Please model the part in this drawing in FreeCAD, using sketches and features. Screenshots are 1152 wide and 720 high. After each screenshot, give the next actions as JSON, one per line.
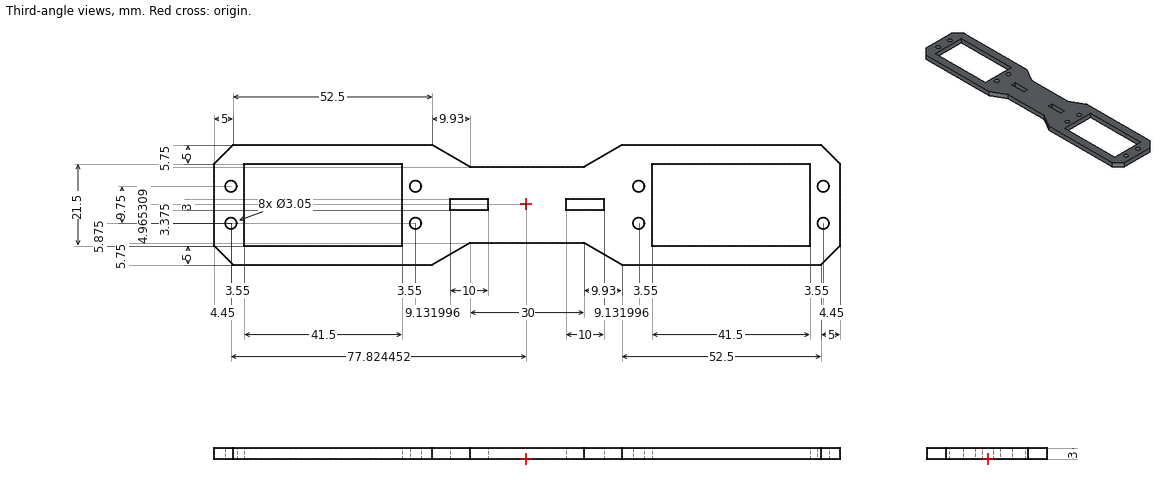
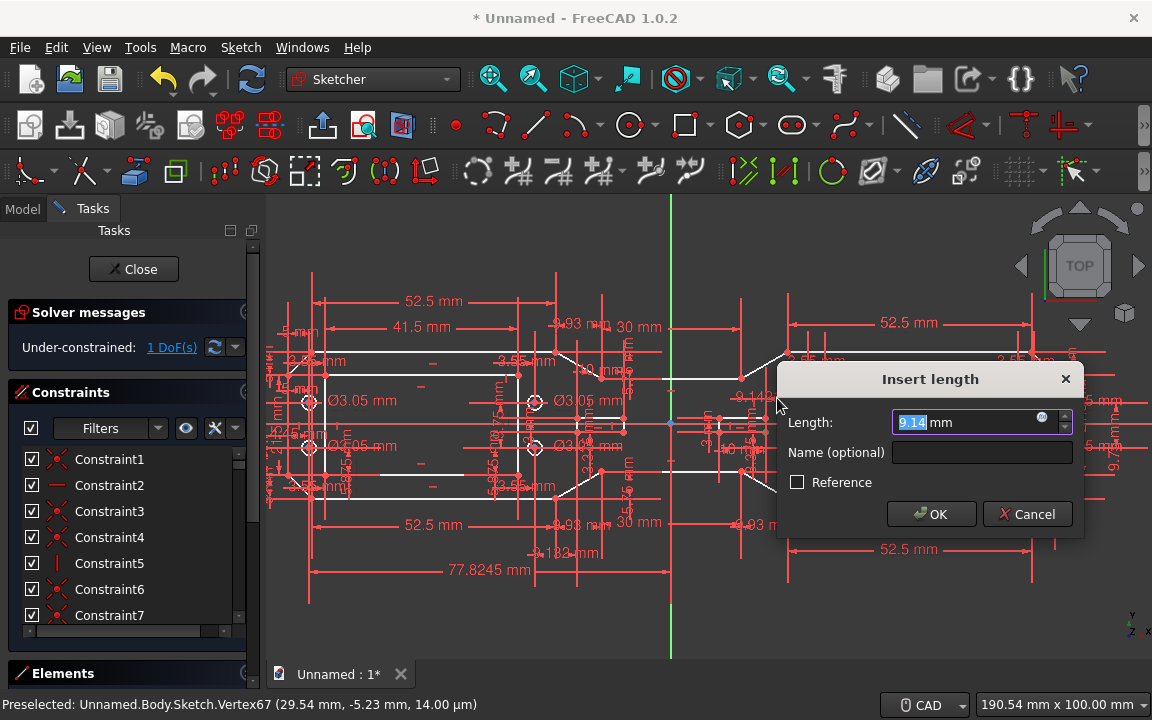
{"action": "type", "text": "9.131996"}
{"action": "key", "text": "Return"}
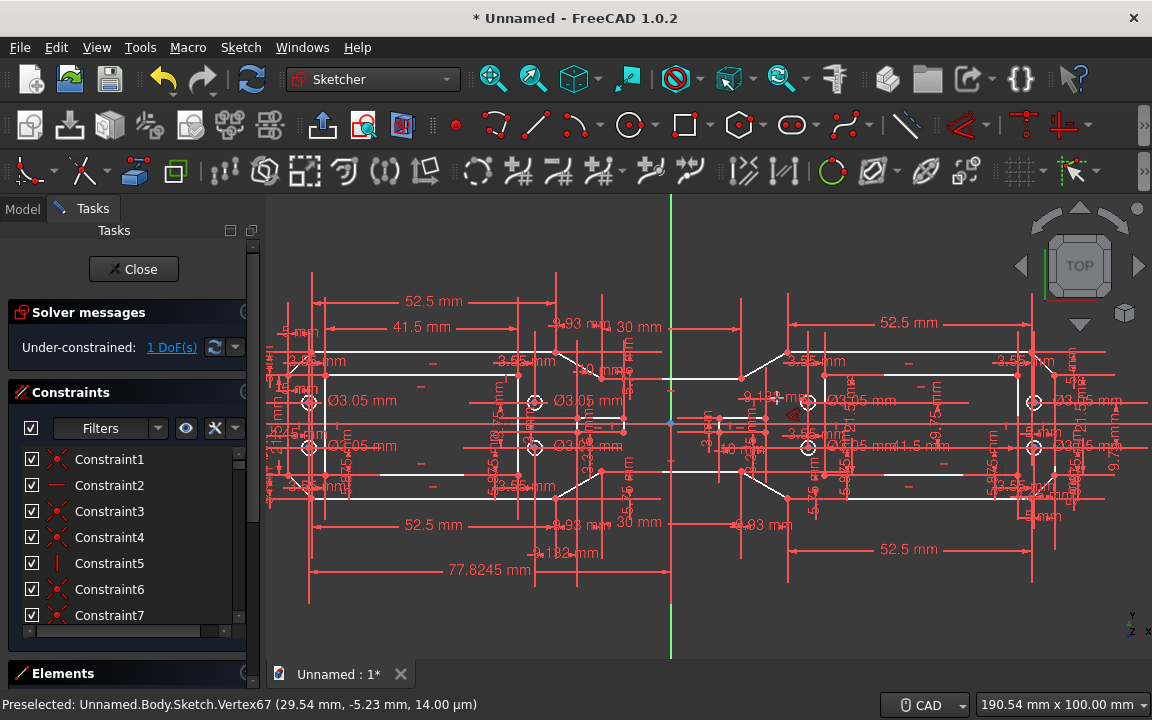
{"action": "scroll", "coordinate": [309, 448], "scroll_direction": "up", "scroll_amount": 3}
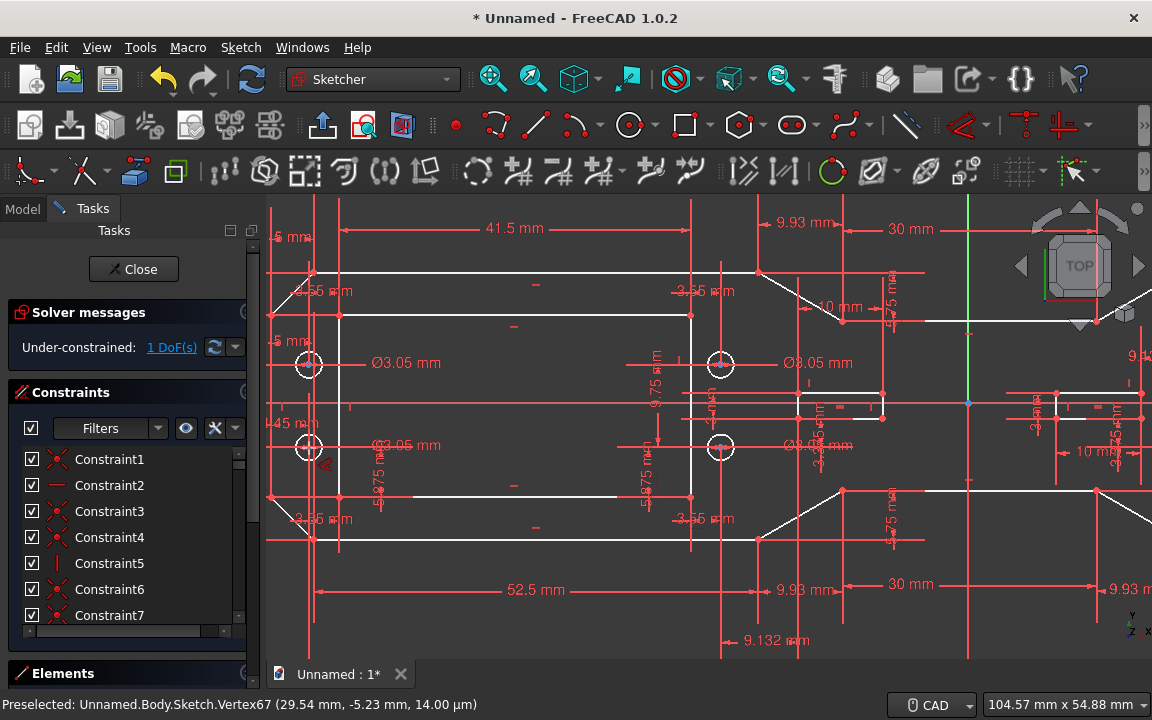
{"action": "left_click", "coordinate": [309, 447]}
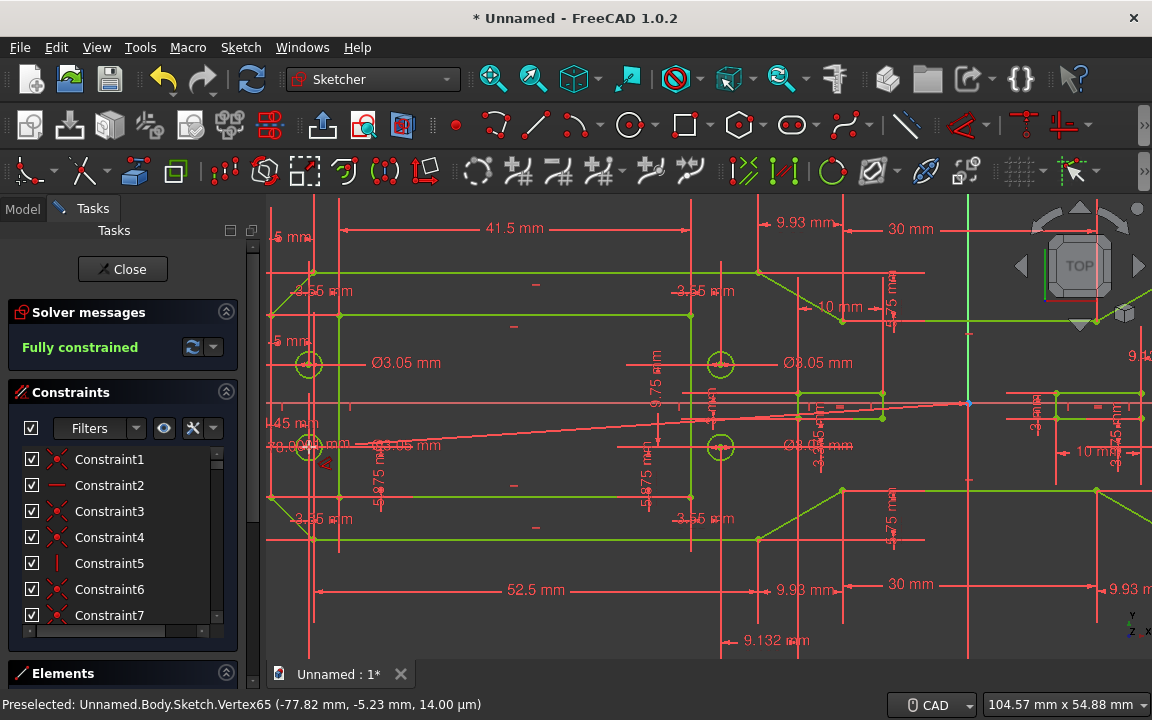
{"action": "key", "text": "Escape"}
{"action": "key", "text": "Escape"}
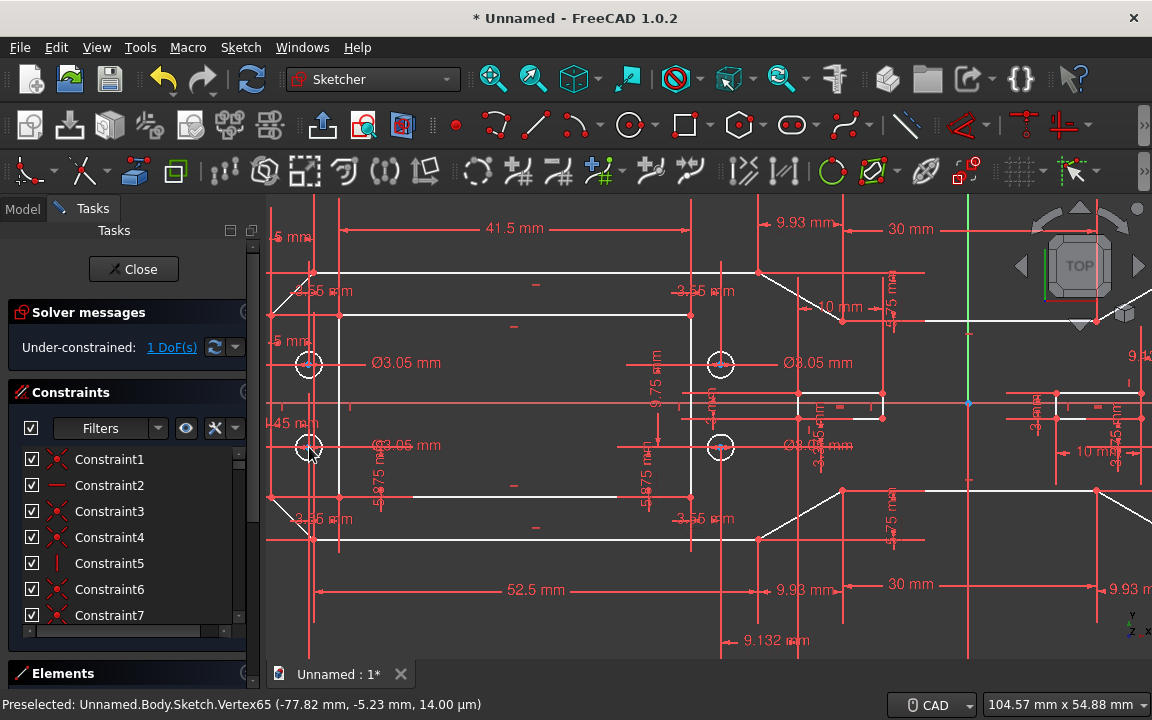
{"action": "left_click", "coordinate": [309, 447]}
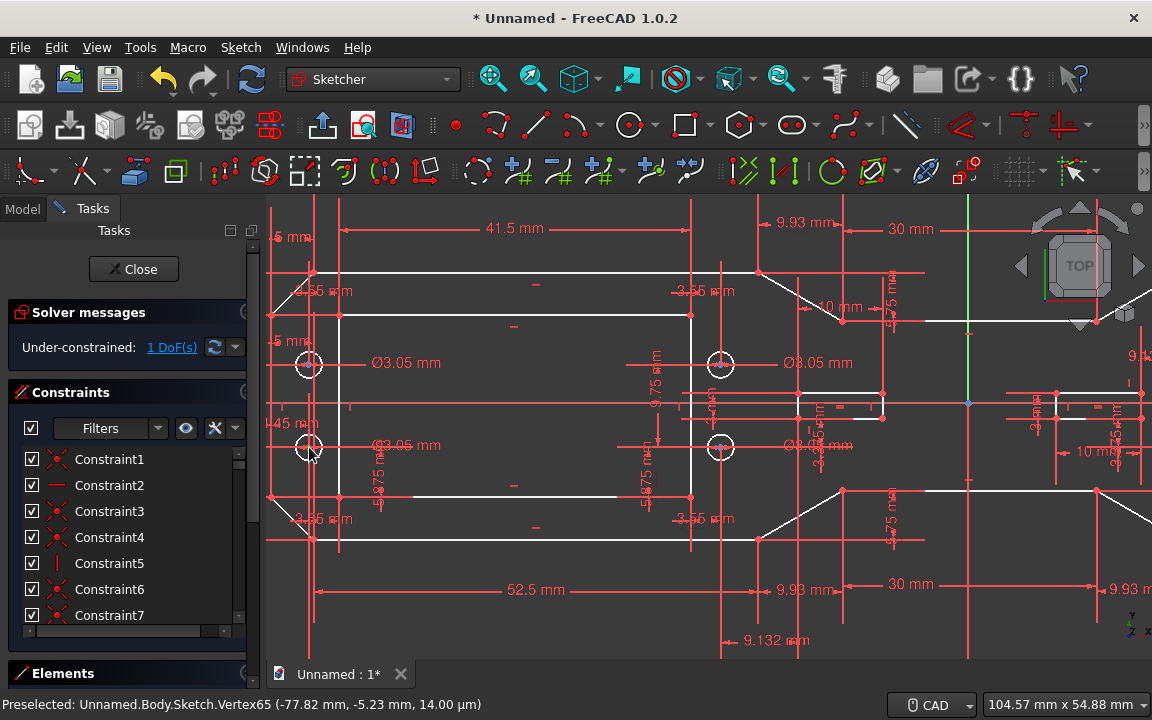
{"action": "left_click", "coordinate": [988, 126]}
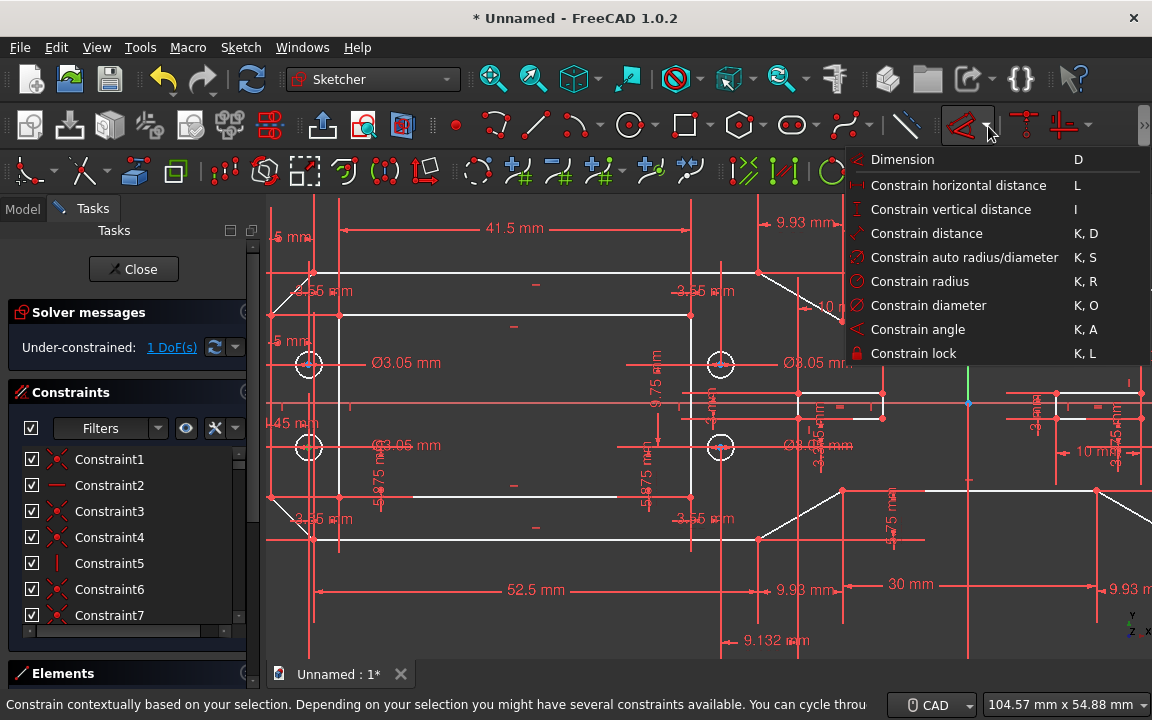
{"action": "left_click", "coordinate": [998, 209]}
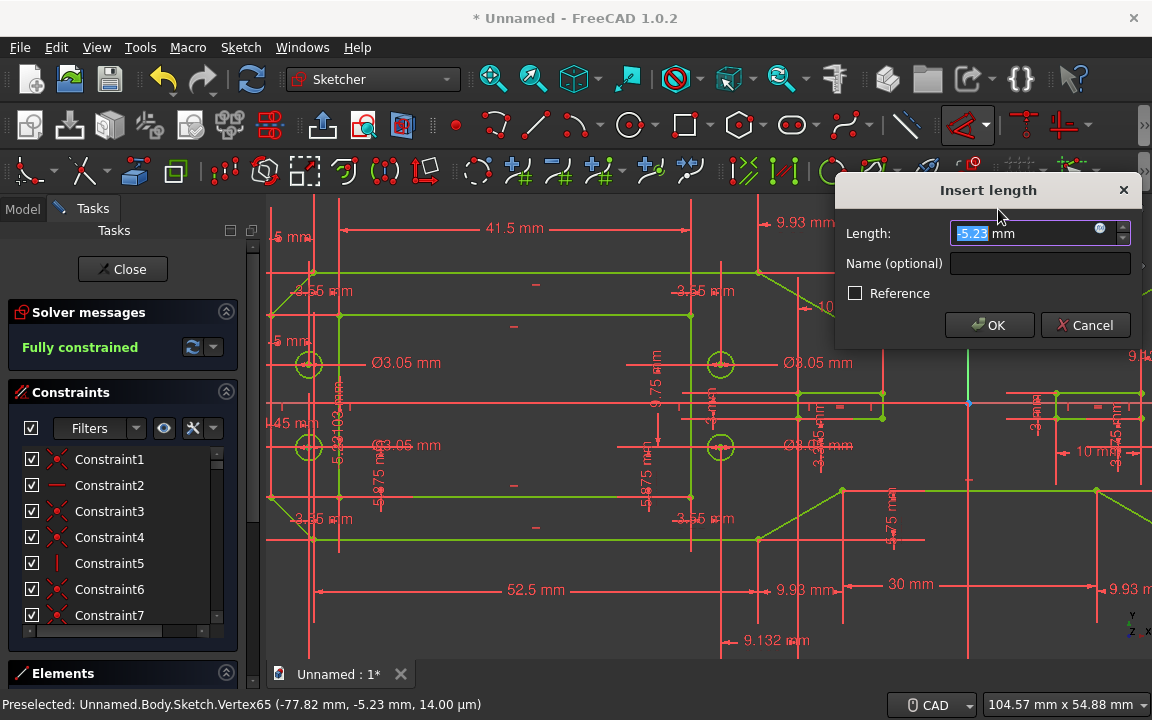
{"action": "type", "text": "-4.965309"}
{"action": "key", "text": "Return"}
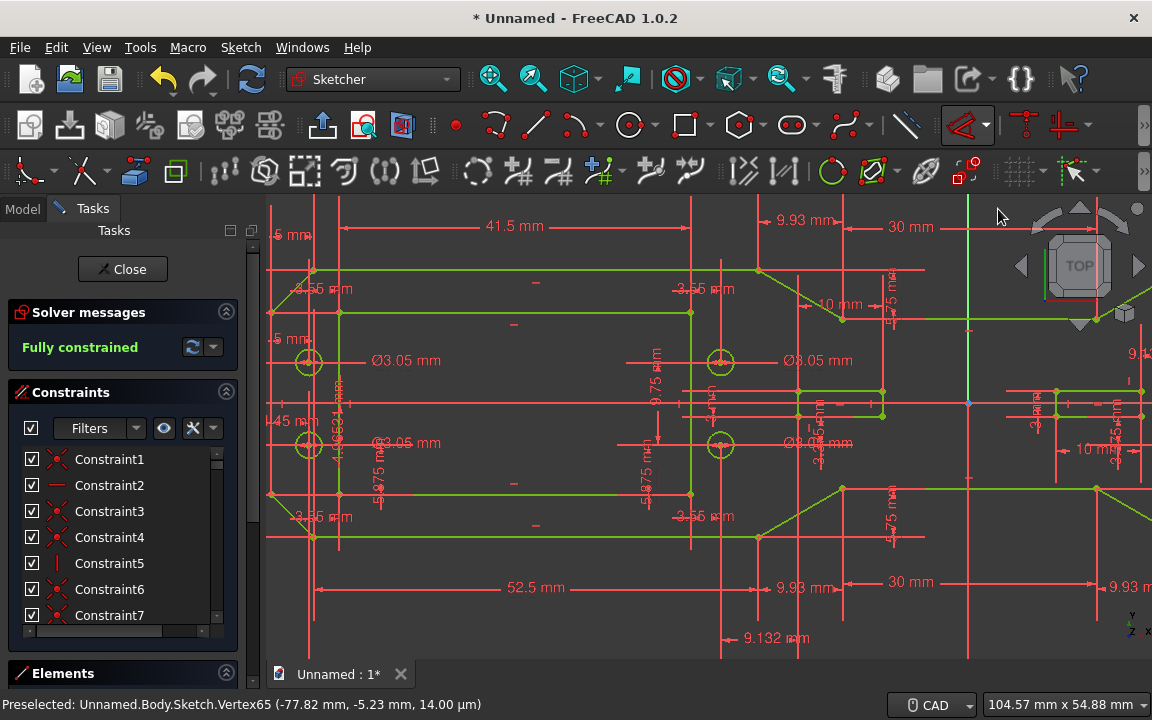
{"action": "left_click", "coordinate": [123, 269]}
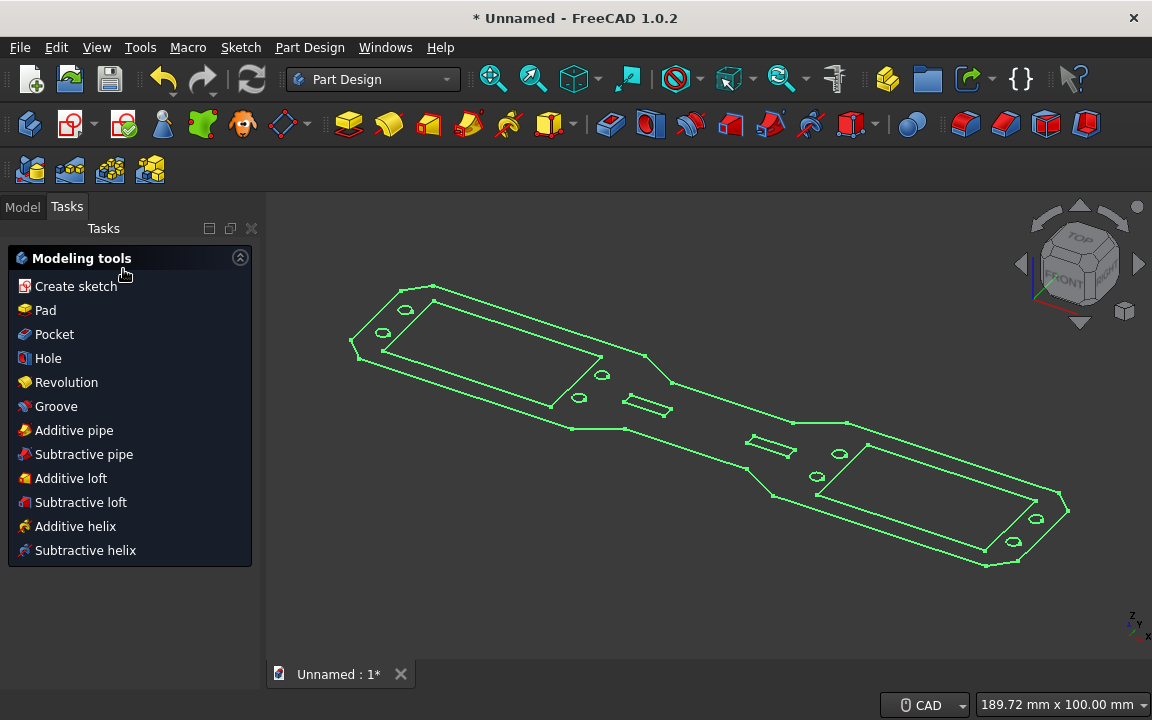
{"action": "left_click", "coordinate": [350, 124]}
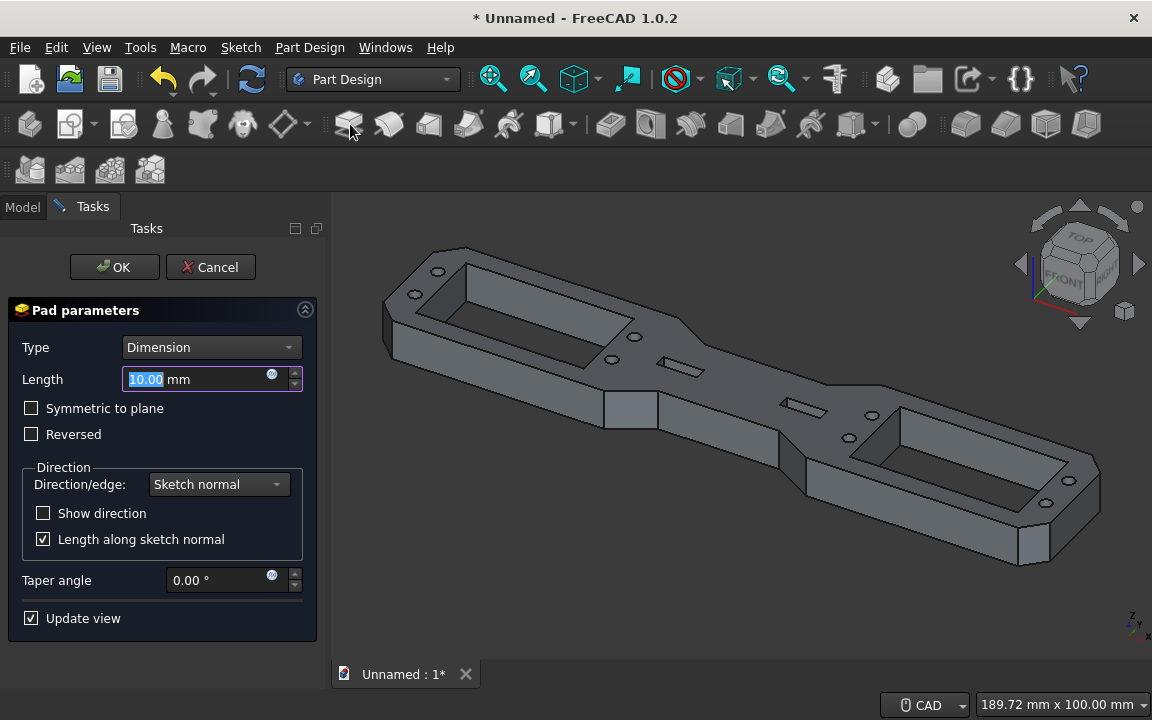
{"action": "type", "text": "3"}
{"action": "key", "text": "Tab"}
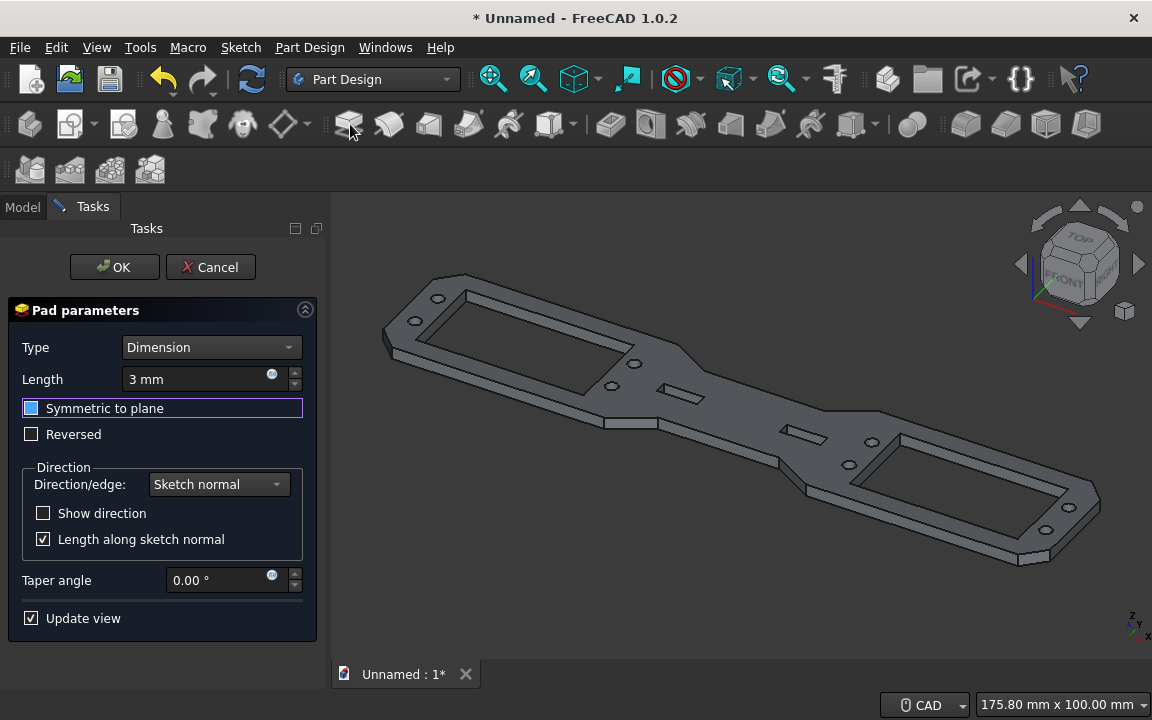
{"action": "left_click", "coordinate": [115, 267]}